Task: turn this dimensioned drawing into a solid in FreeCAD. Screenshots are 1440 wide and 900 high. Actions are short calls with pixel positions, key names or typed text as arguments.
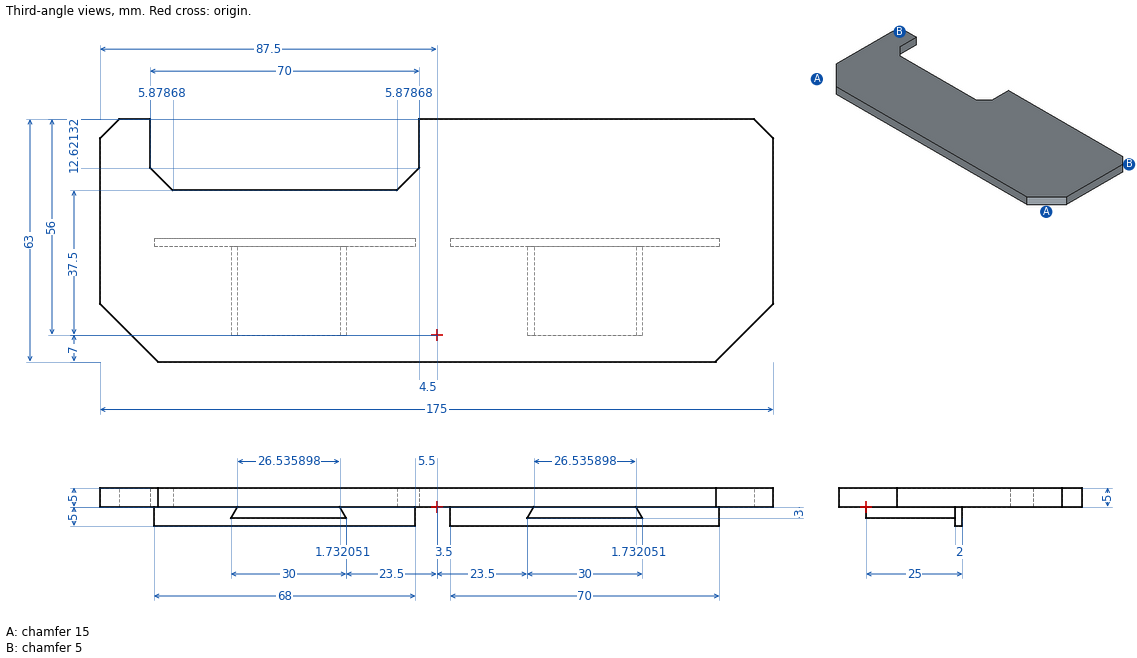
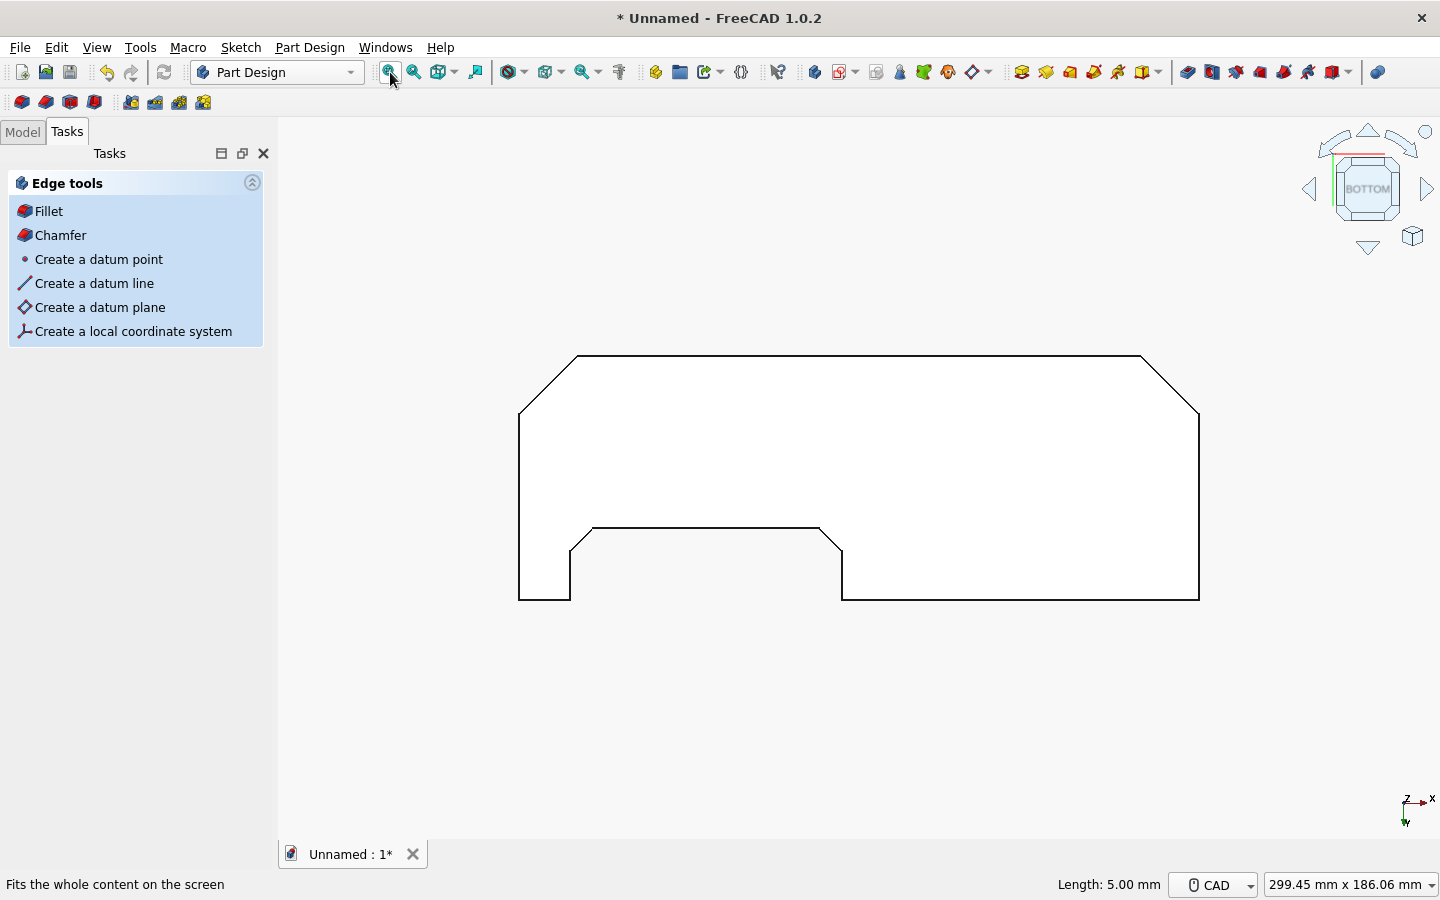
scroll(519, 599, up, 4)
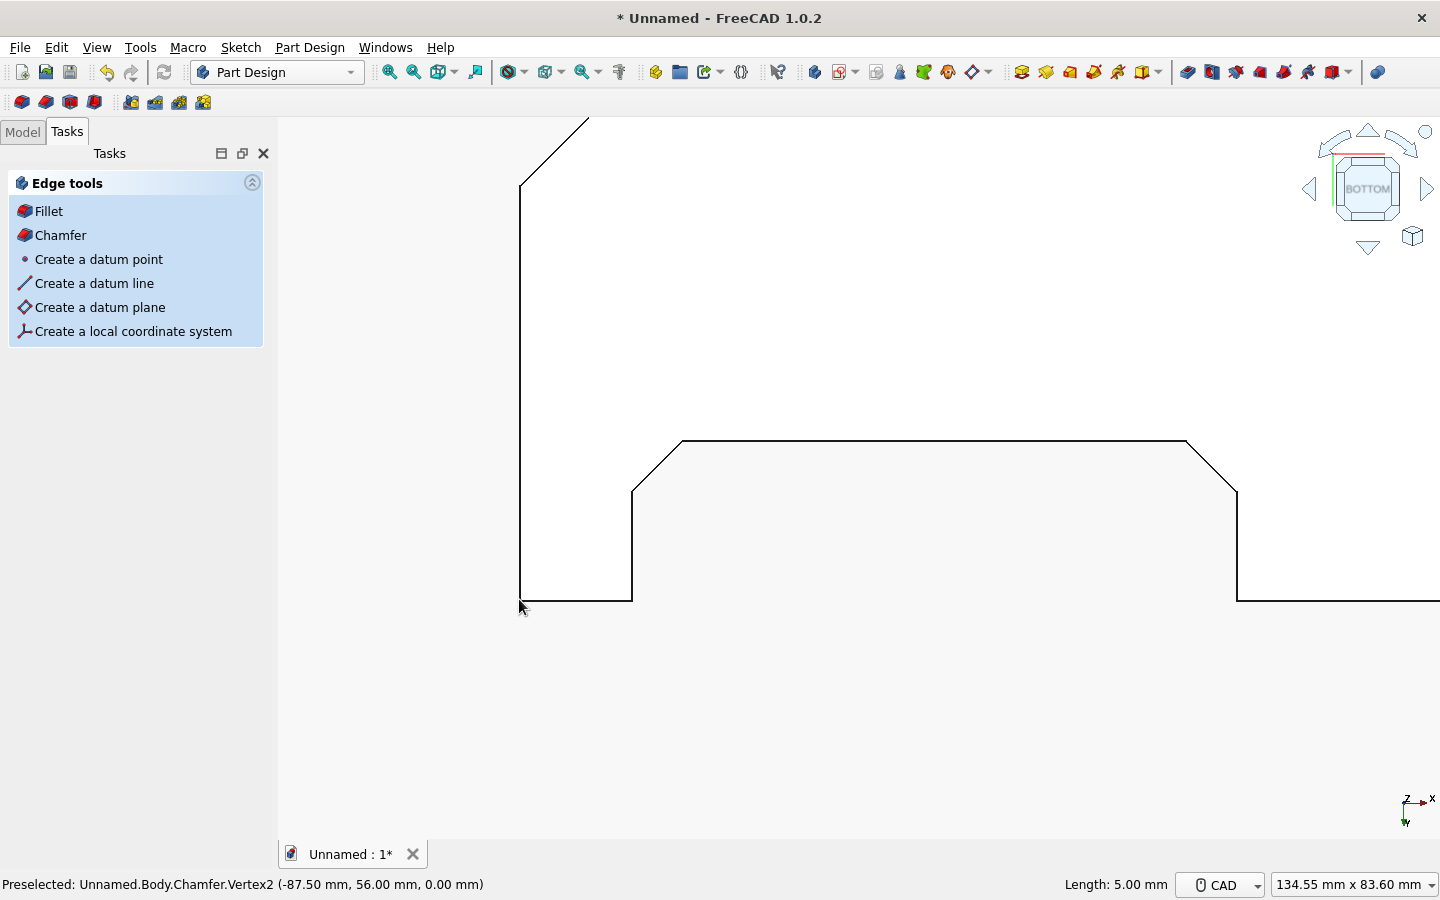
click(390, 72)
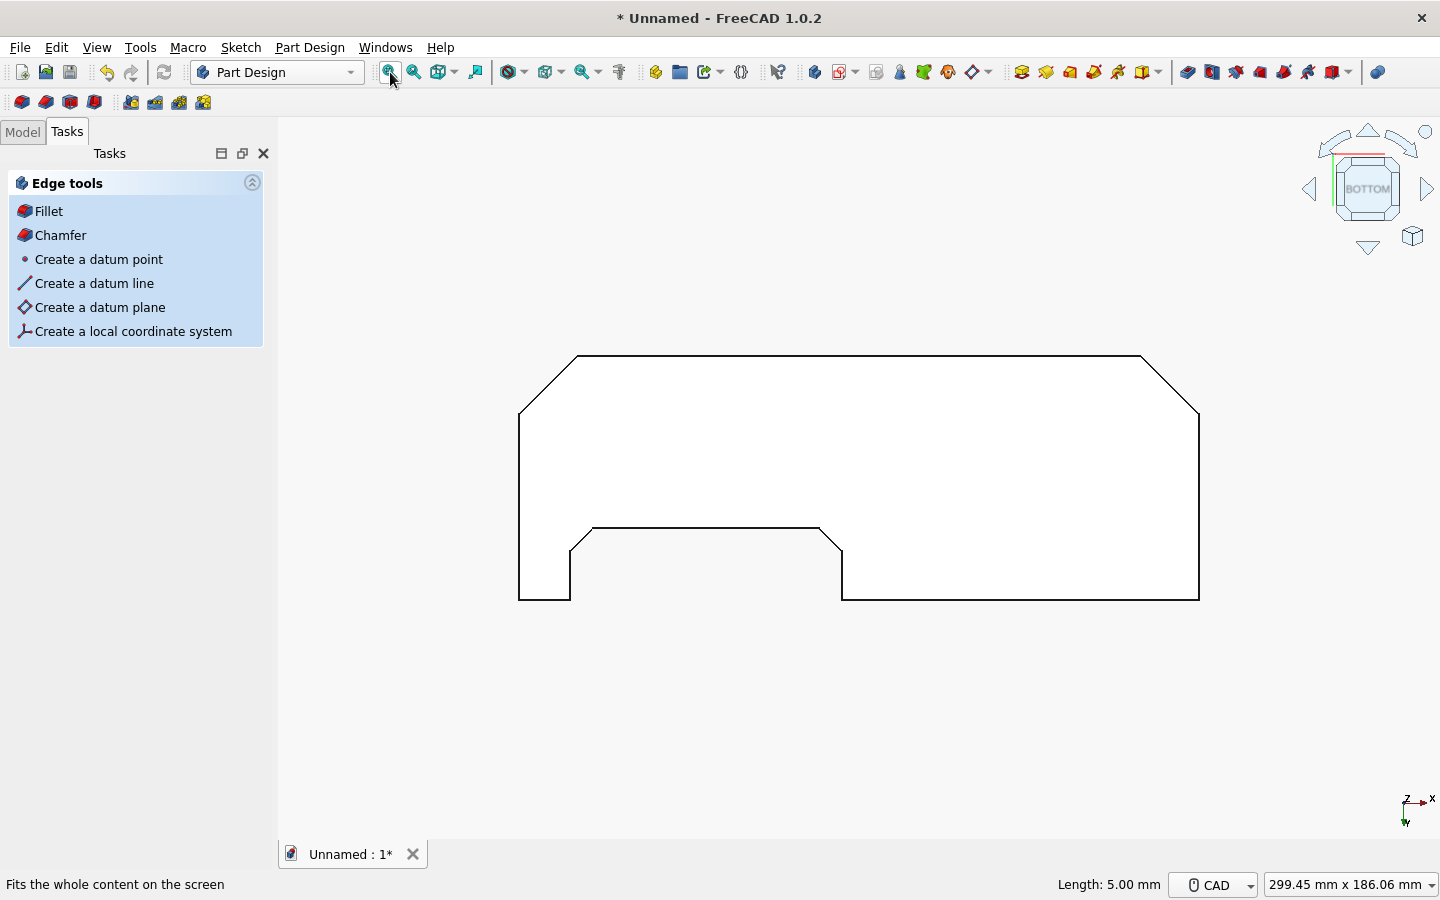
key(4)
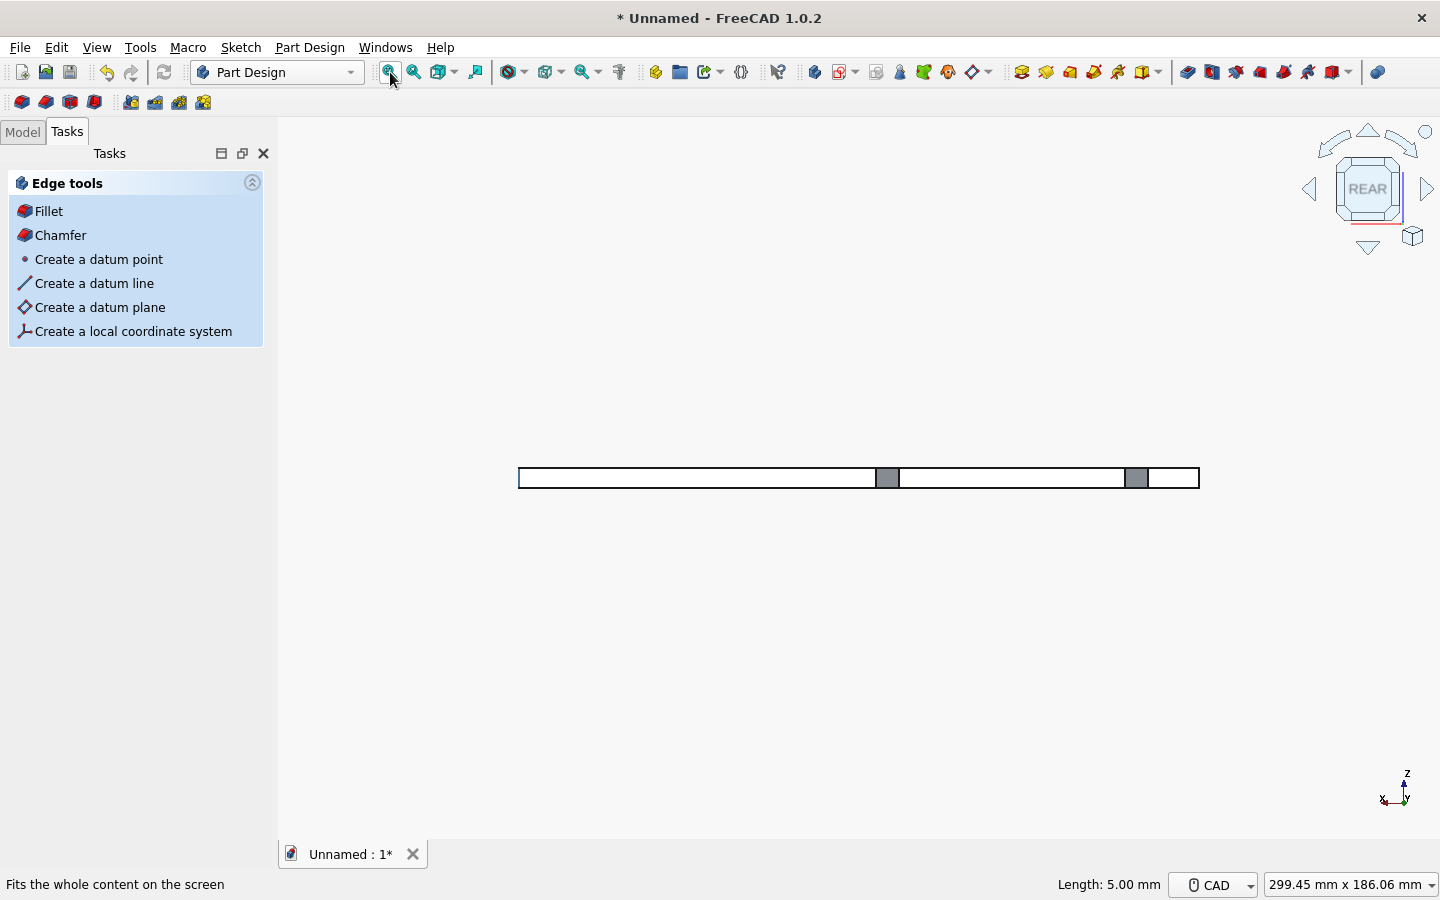
click(1199, 477, ctrl)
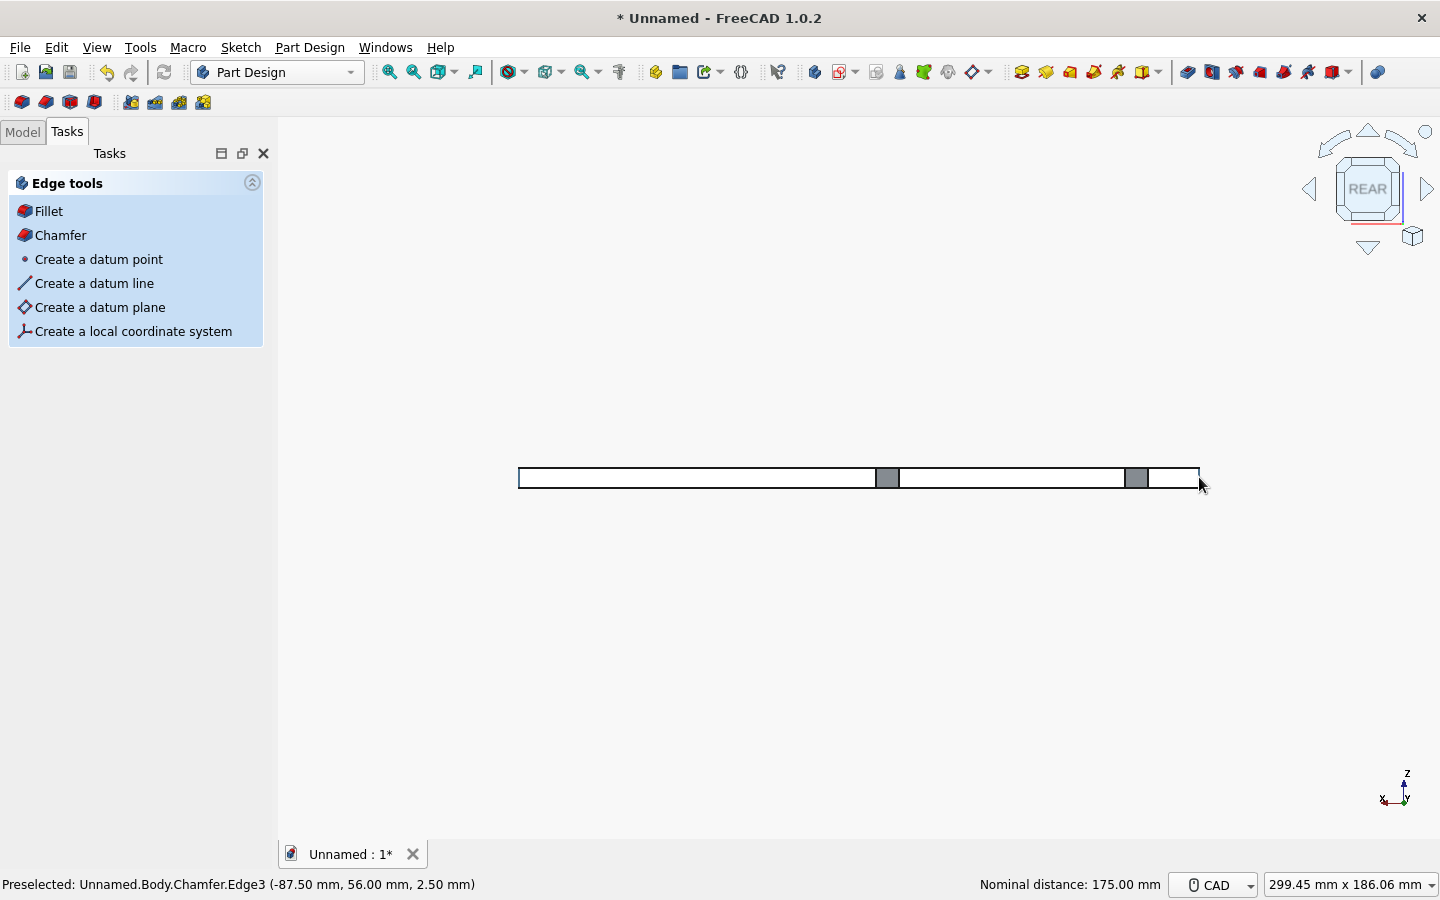
click(46, 102)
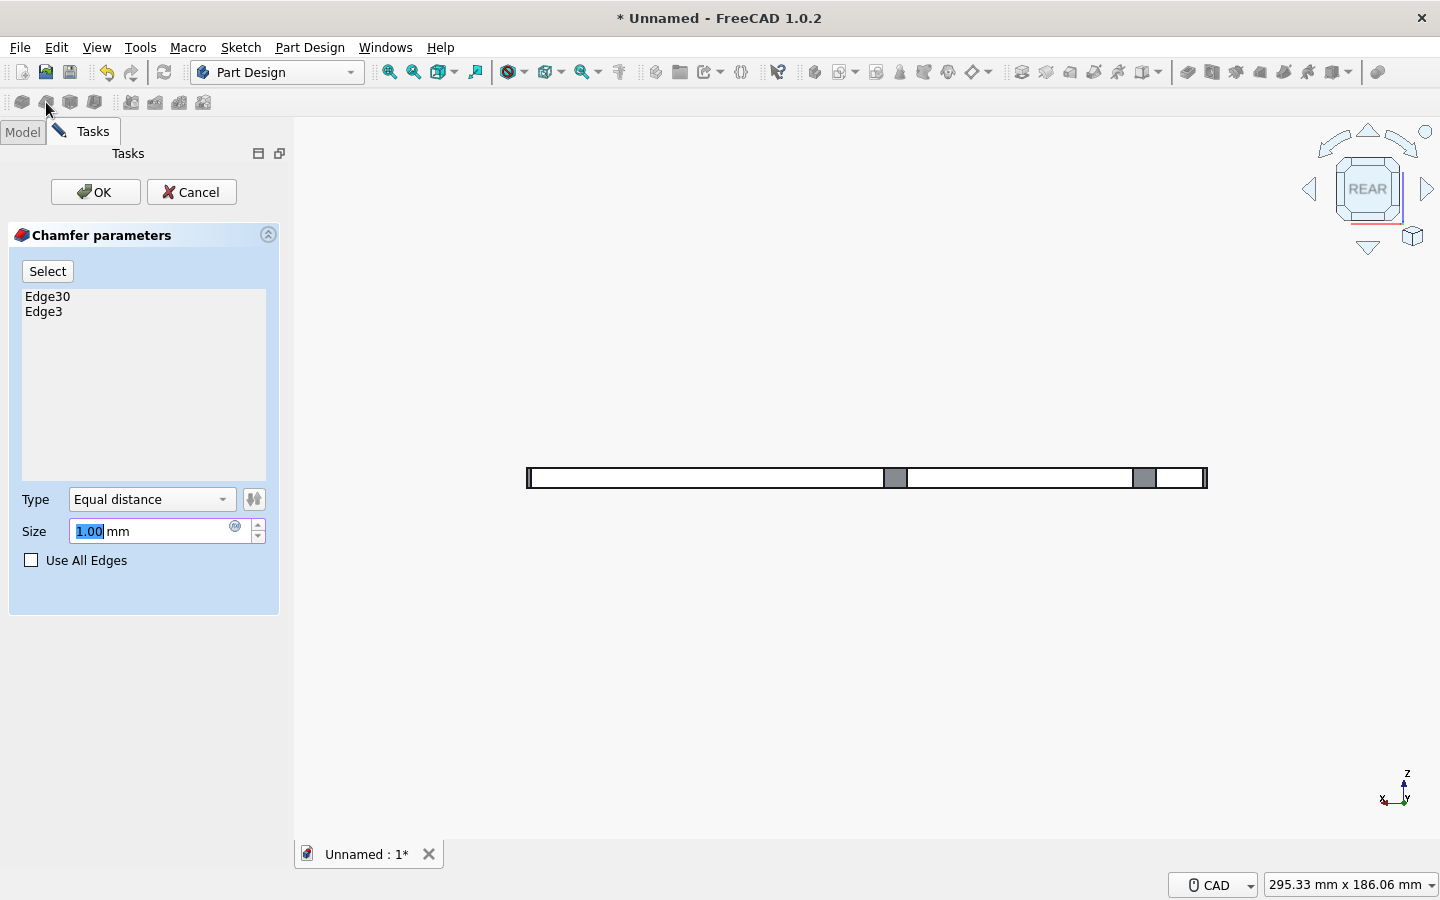
text(5)
key(Tab)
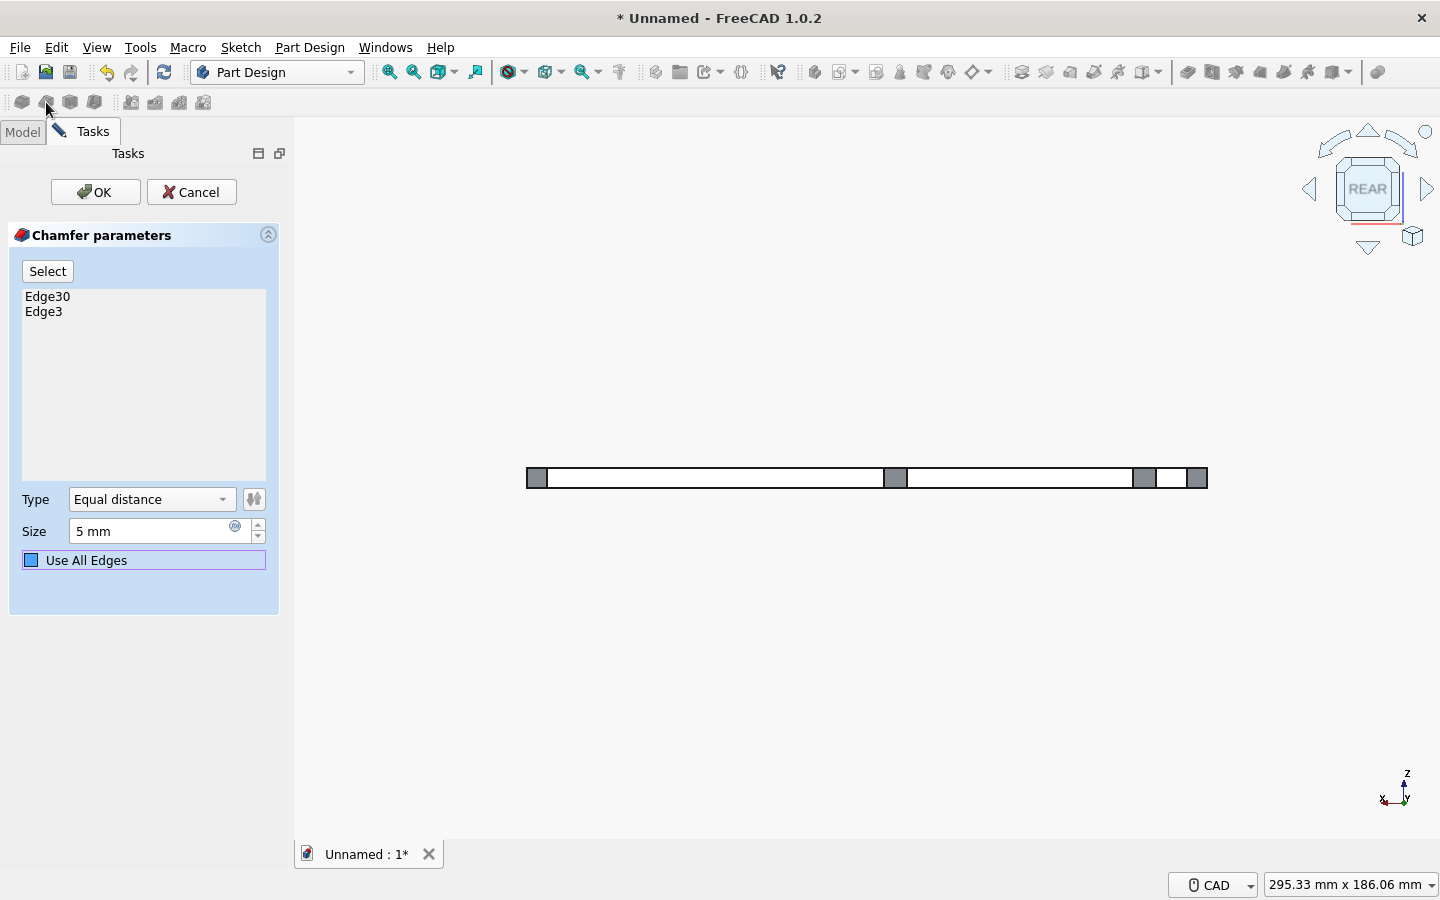
click(96, 192)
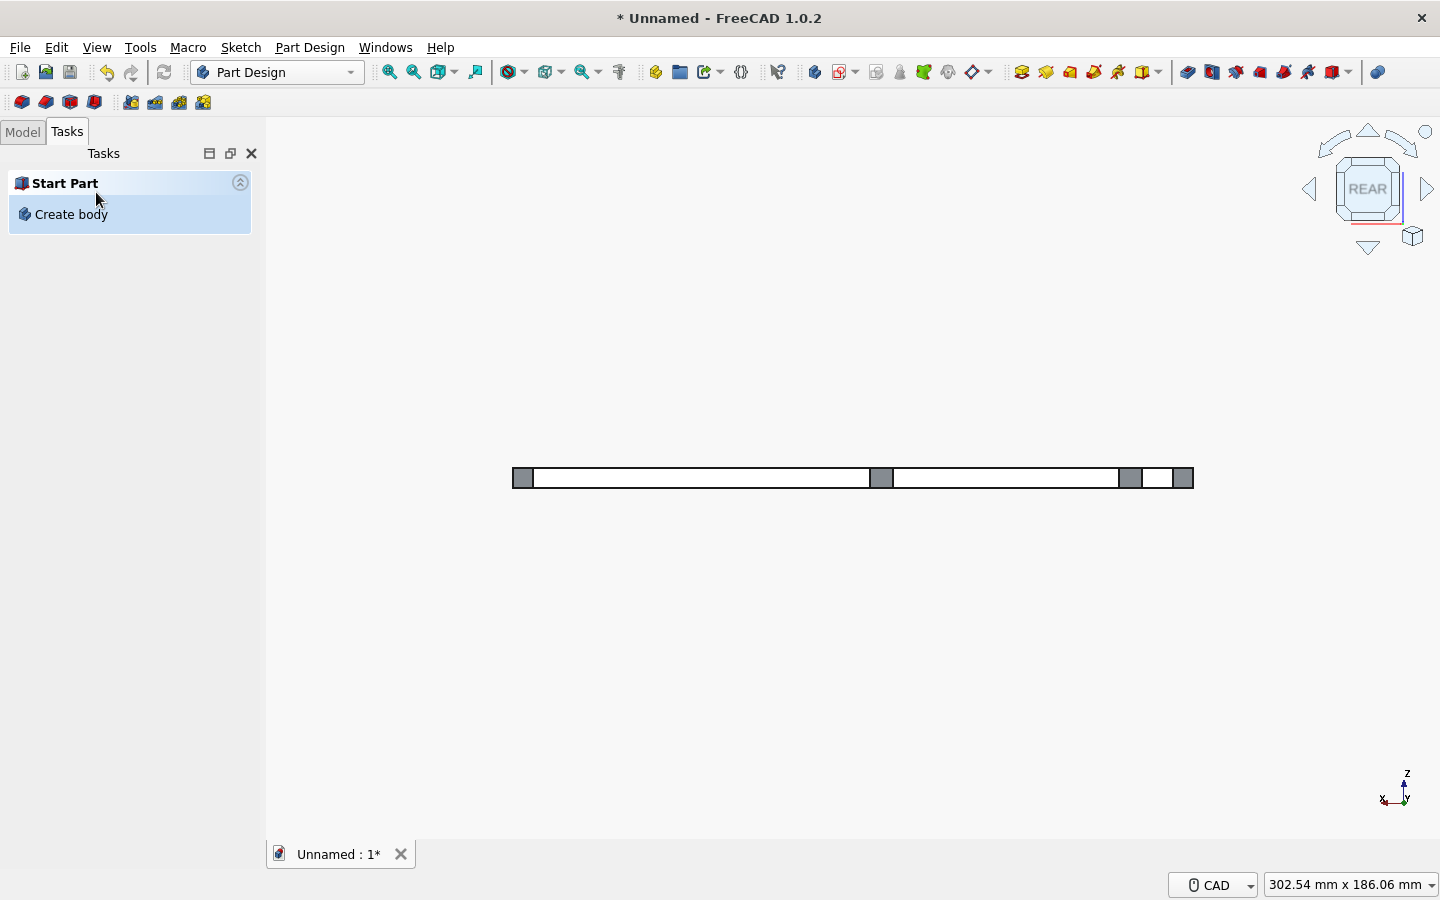
click(840, 72)